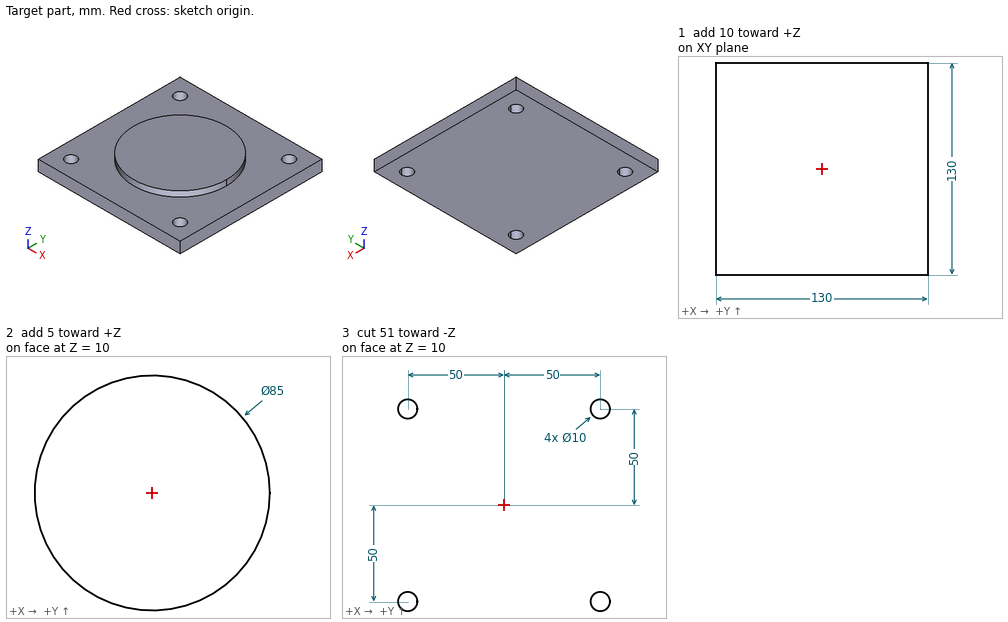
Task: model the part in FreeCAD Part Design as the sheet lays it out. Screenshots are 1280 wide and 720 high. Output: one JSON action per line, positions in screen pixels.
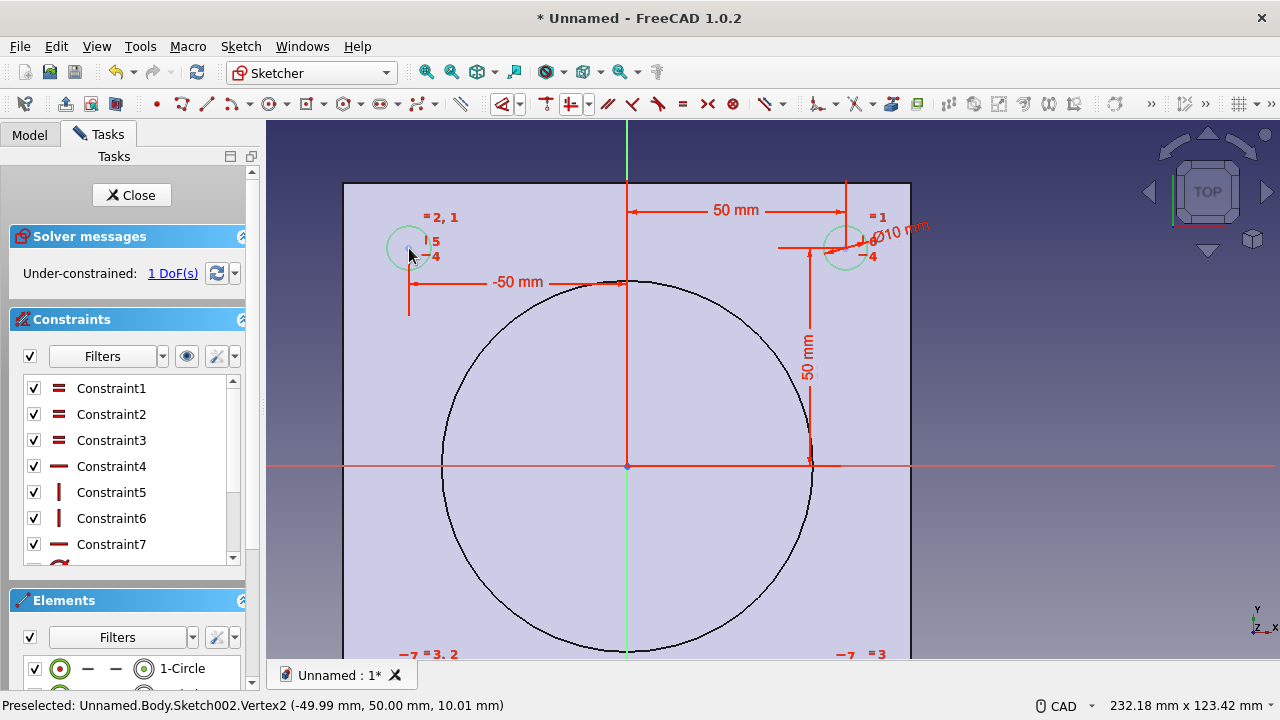
{"action": "scroll", "coordinate": [862, 233], "scroll_direction": "down", "scroll_amount": 2}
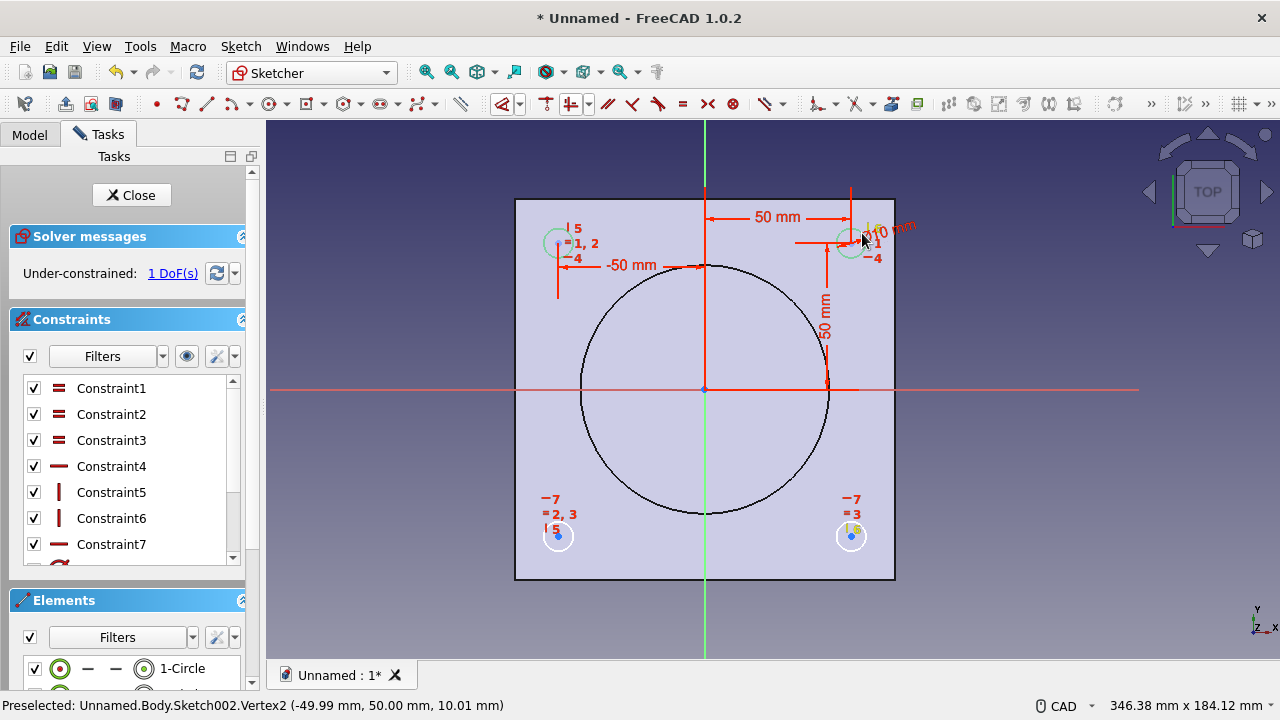
{"action": "left_click", "coordinate": [558, 536]}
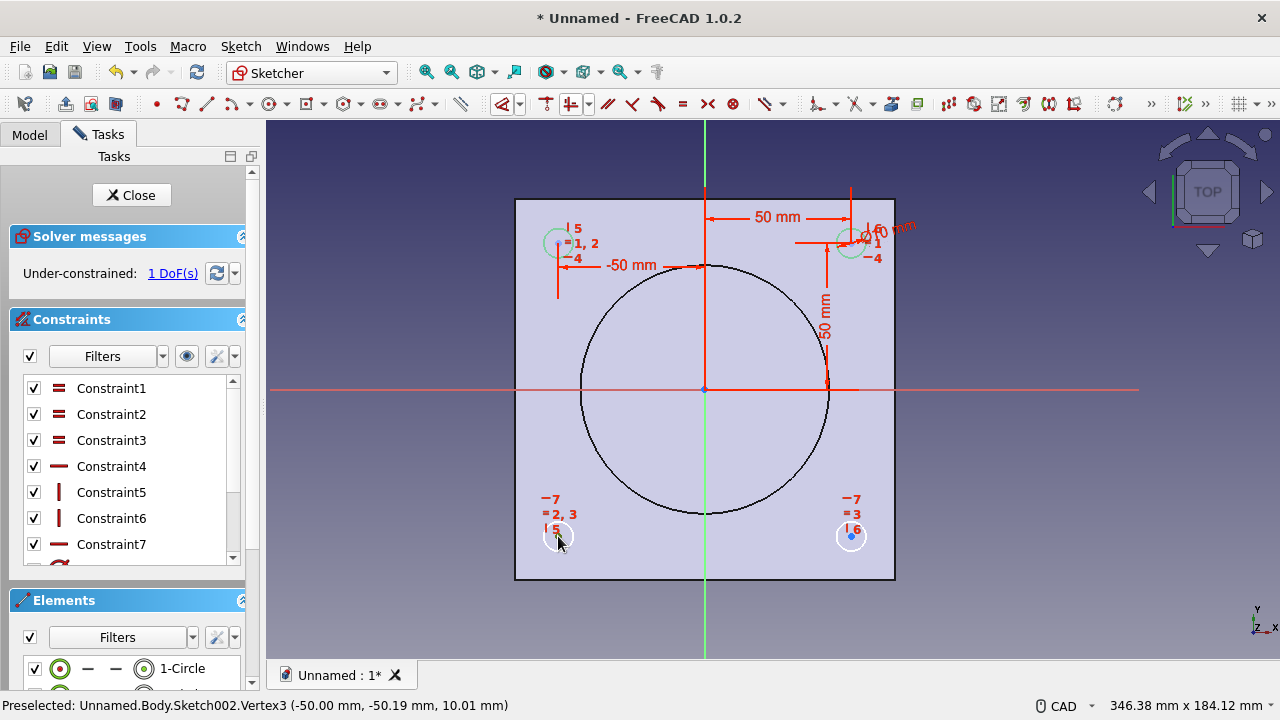
{"action": "left_click", "coordinate": [520, 104]}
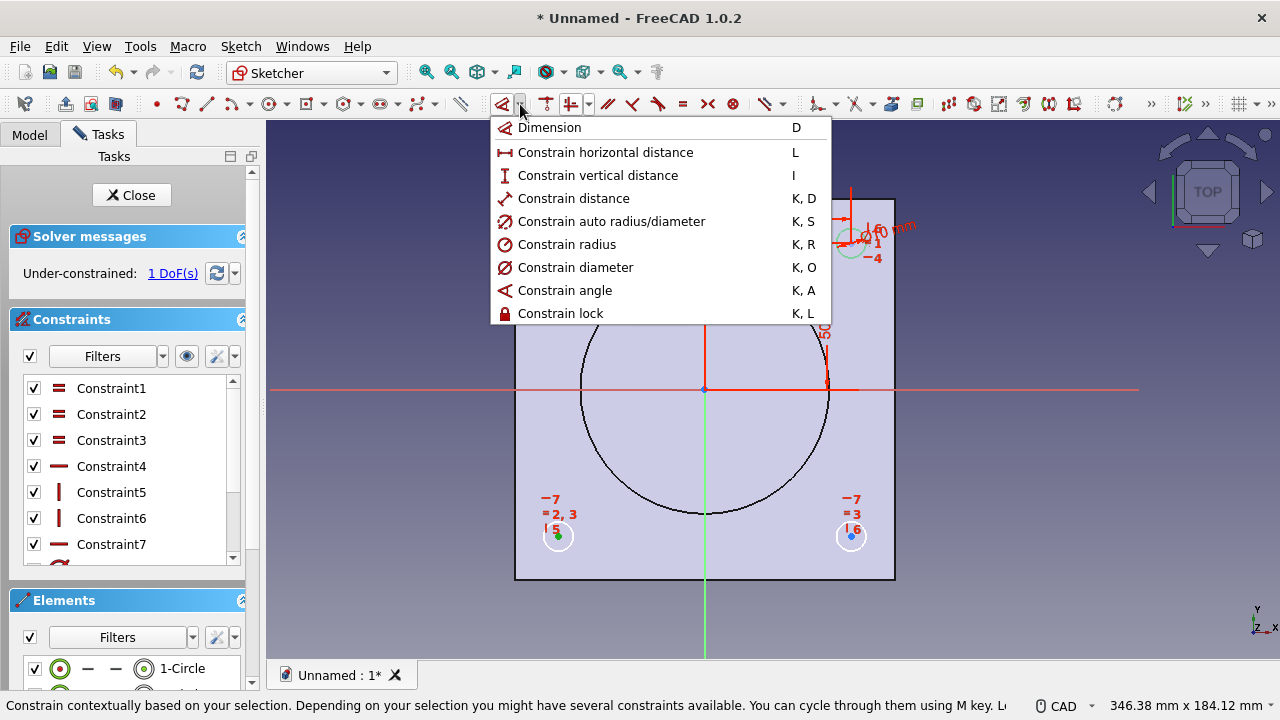
{"action": "left_click", "coordinate": [661, 176]}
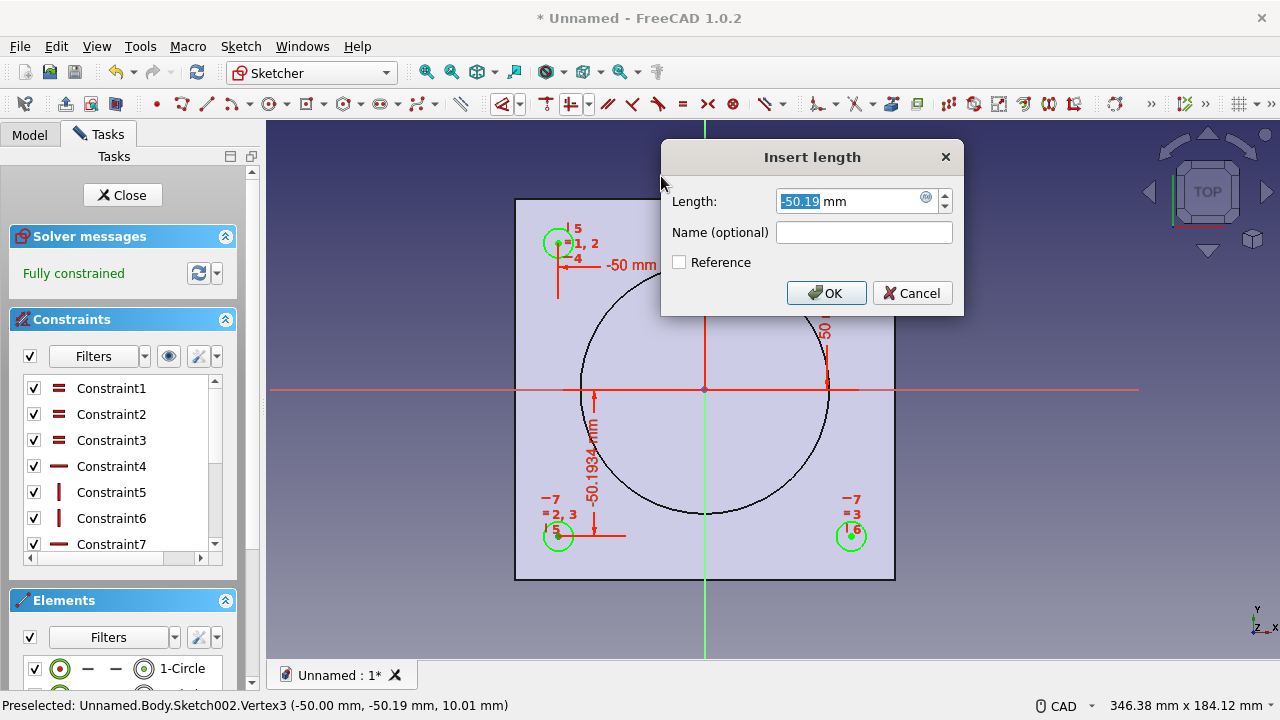
{"action": "type", "text": "-50"}
{"action": "key", "text": "Return"}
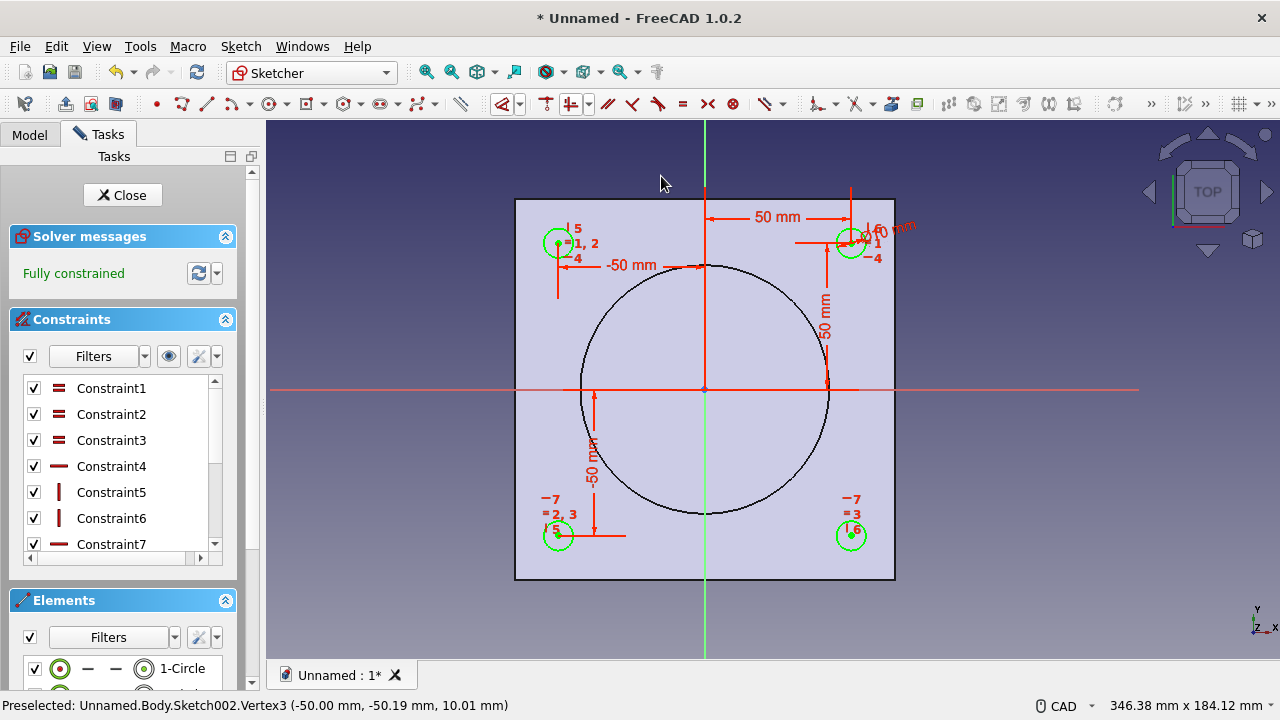
{"action": "left_click", "coordinate": [123, 195]}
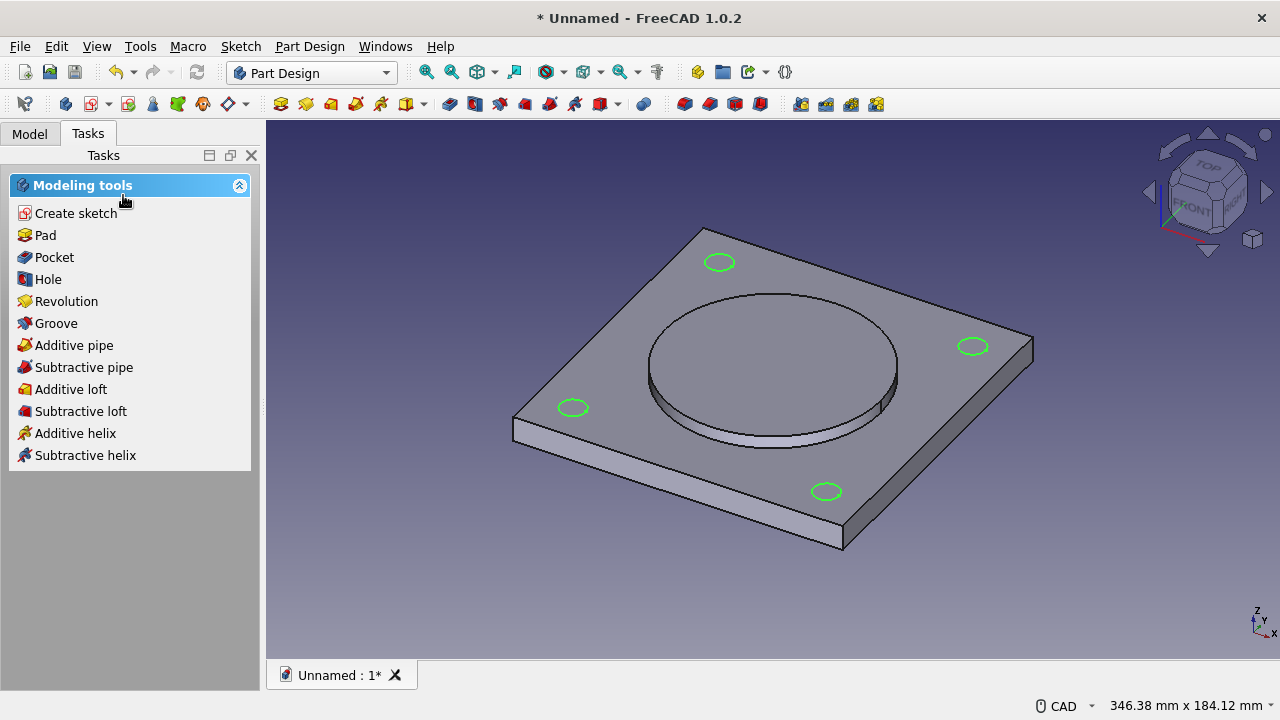
{"action": "left_click", "coordinate": [450, 104]}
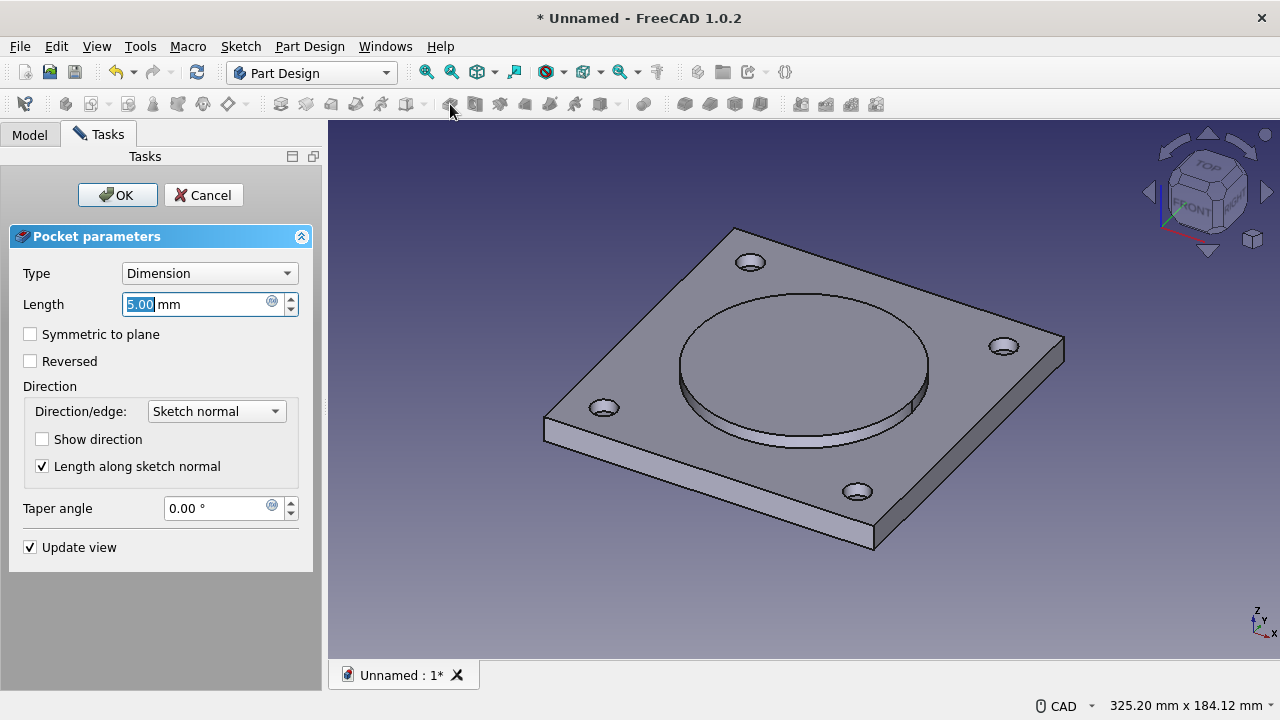
{"action": "type", "text": "51"}
{"action": "key", "text": "Tab"}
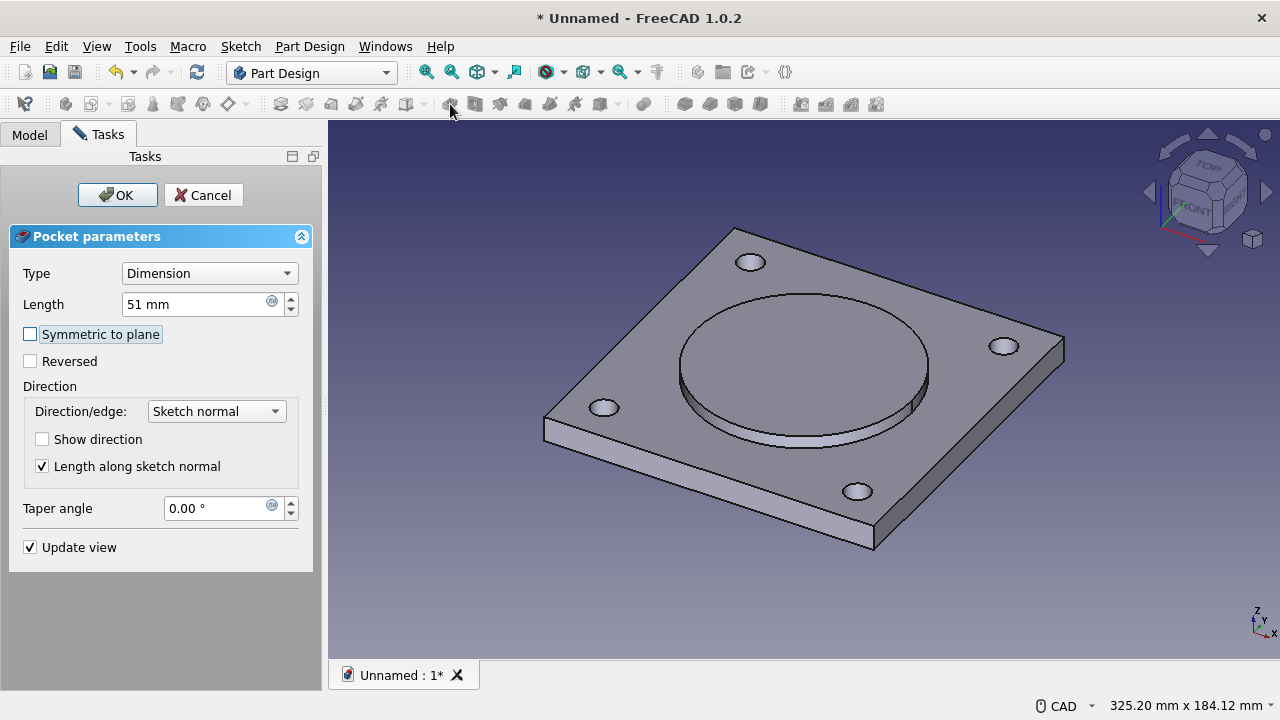
{"action": "left_click", "coordinate": [118, 195]}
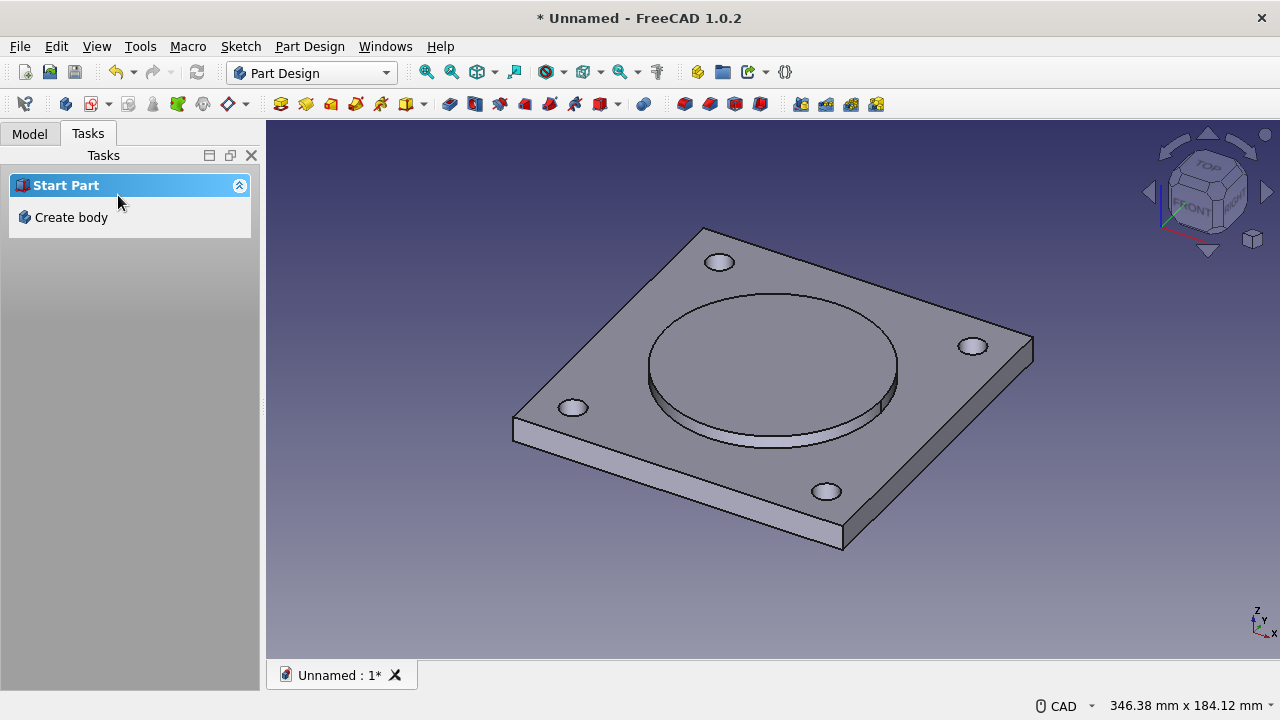
{"action": "key", "text": "0"}